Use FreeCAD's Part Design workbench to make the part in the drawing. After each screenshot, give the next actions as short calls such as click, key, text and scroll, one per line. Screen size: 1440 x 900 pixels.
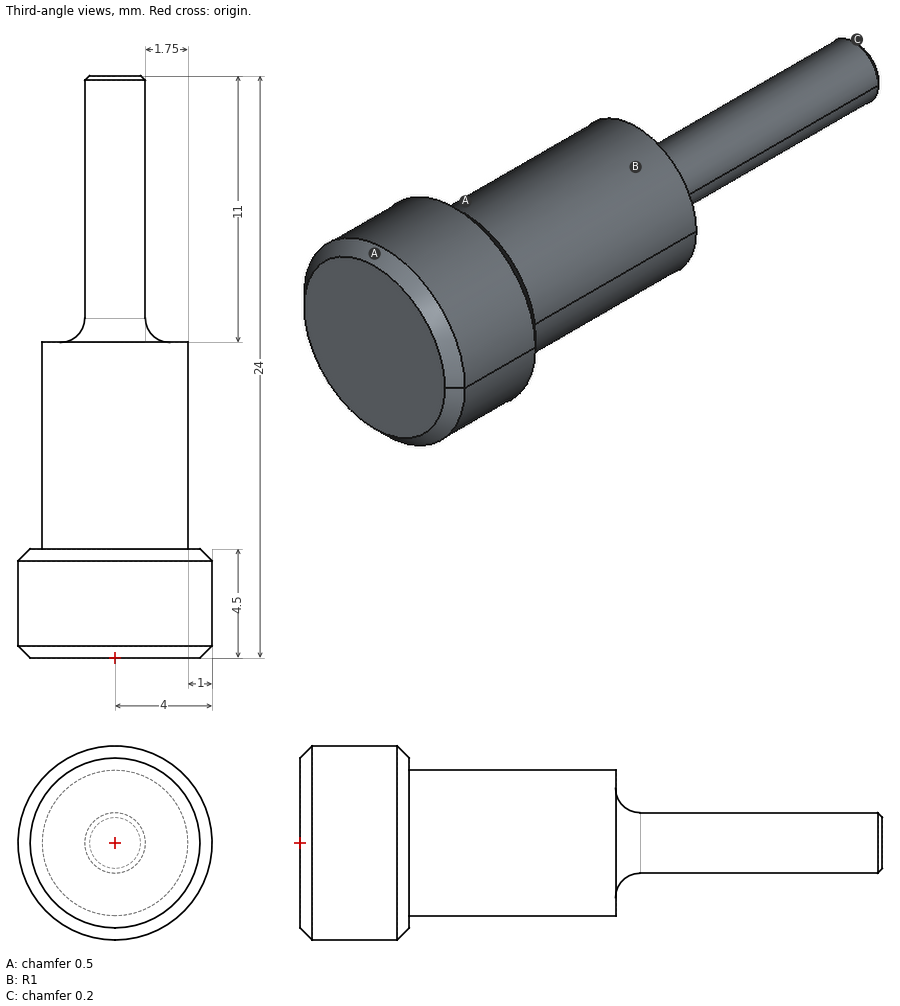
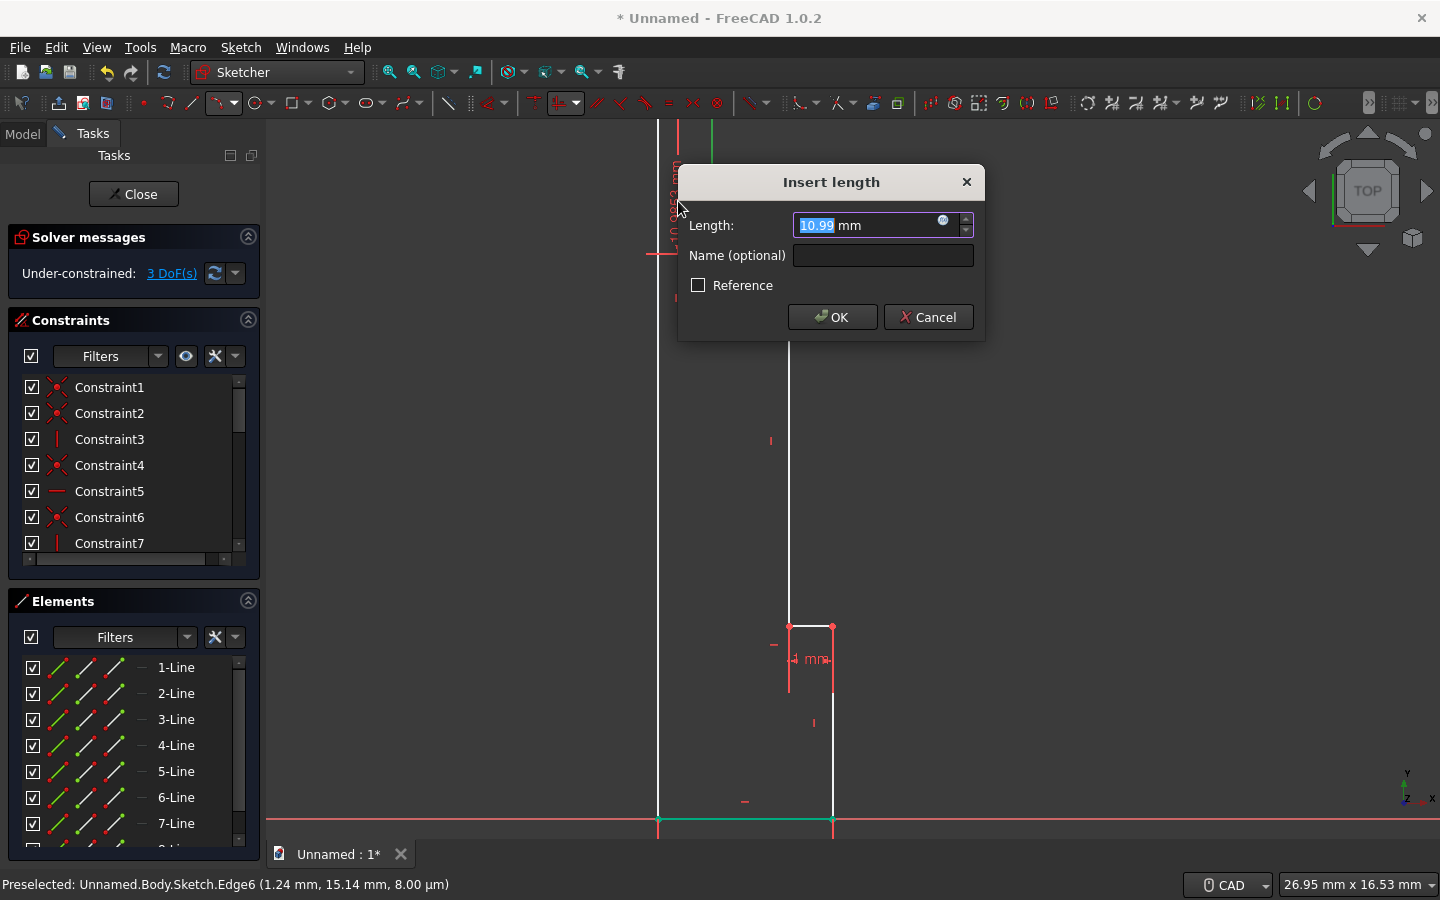
text(11)
key(Return)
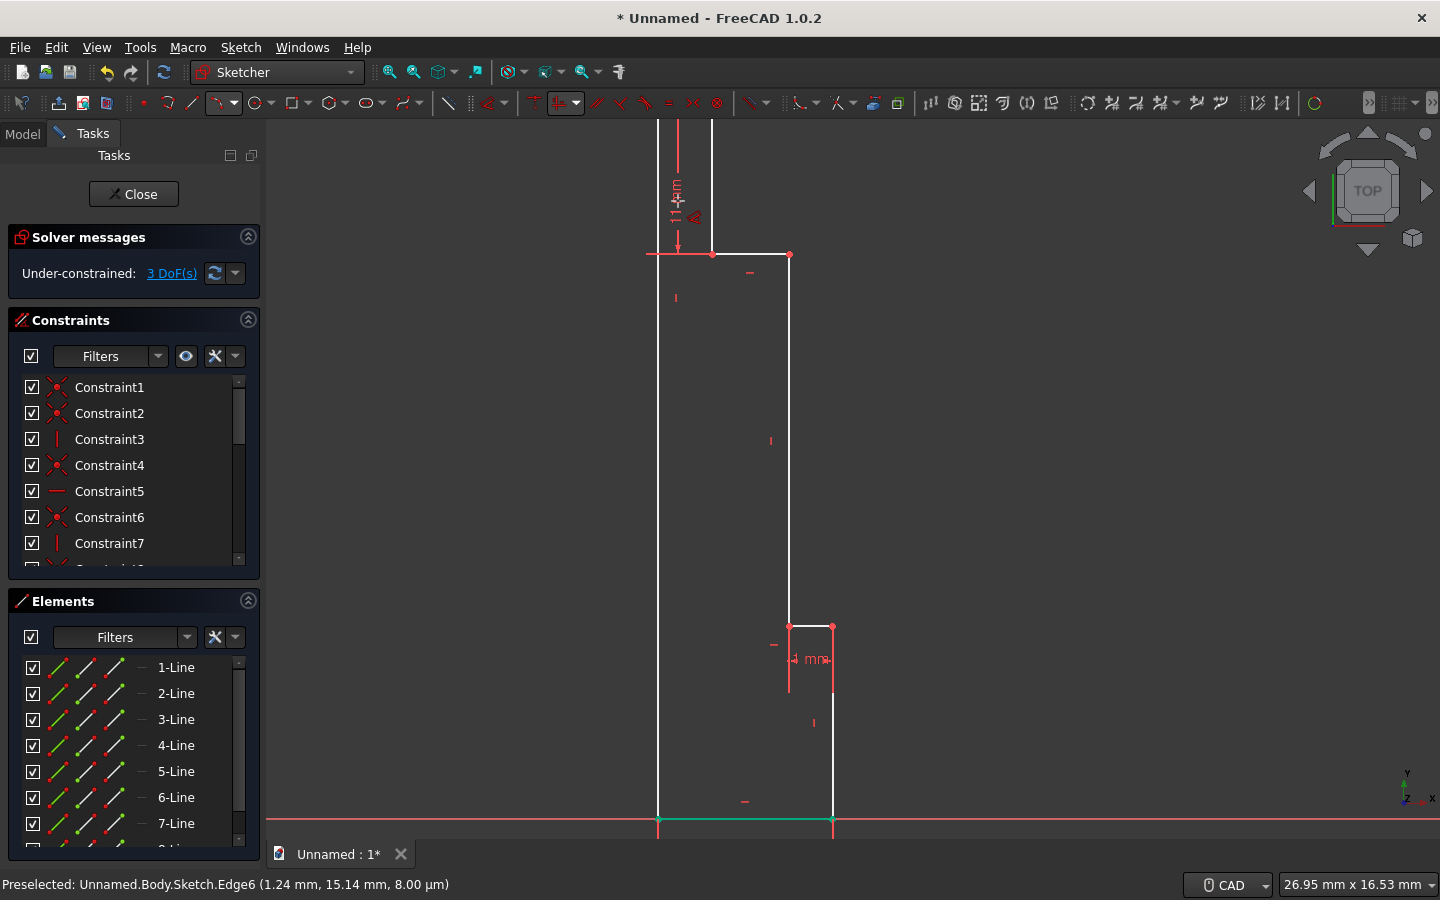
click(658, 506)
click(624, 479)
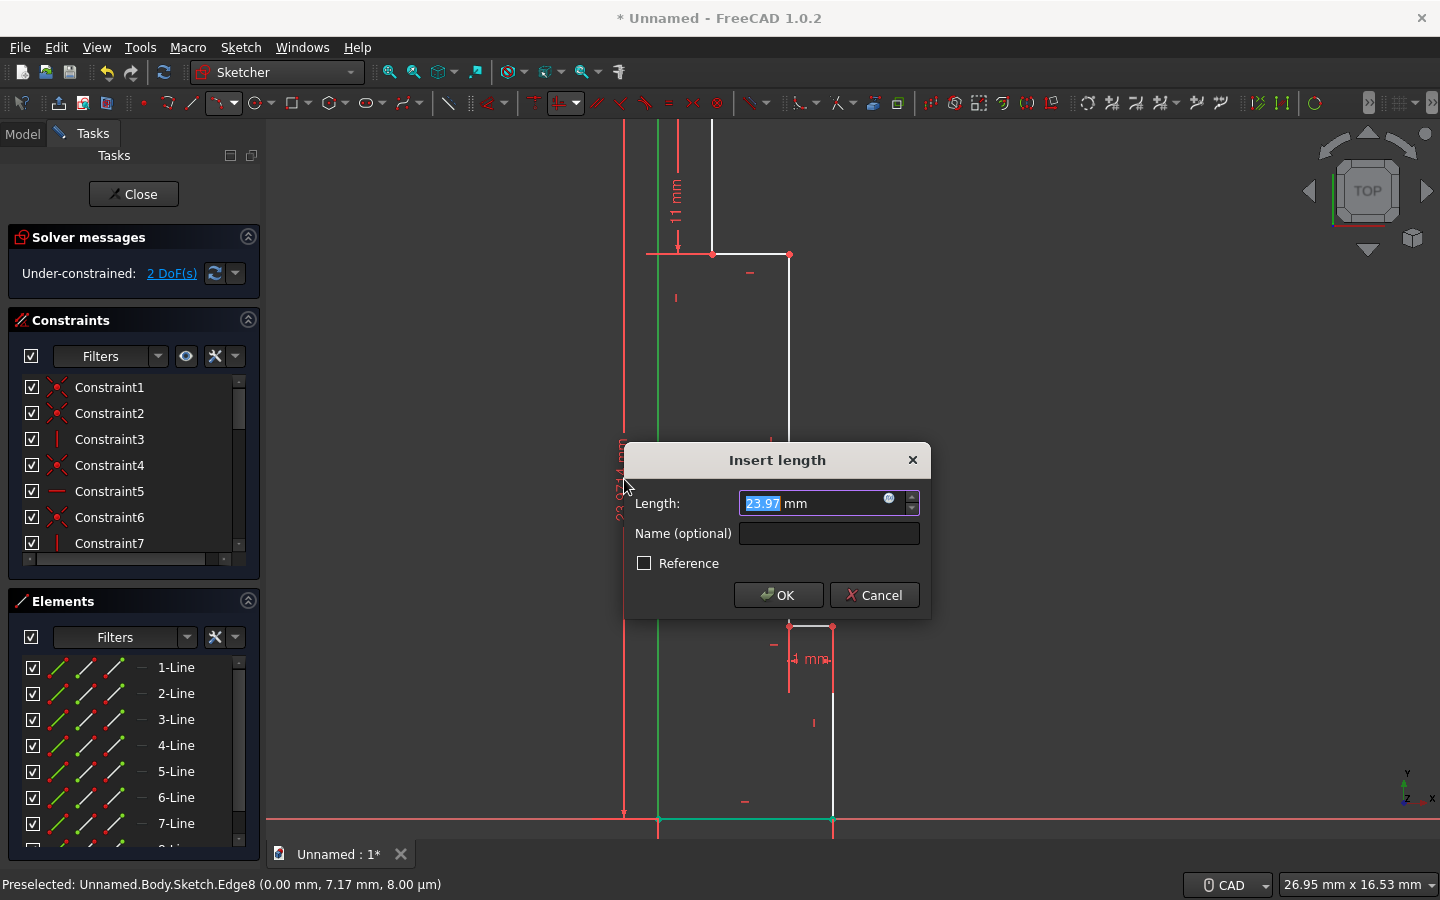
text(24)
key(Return)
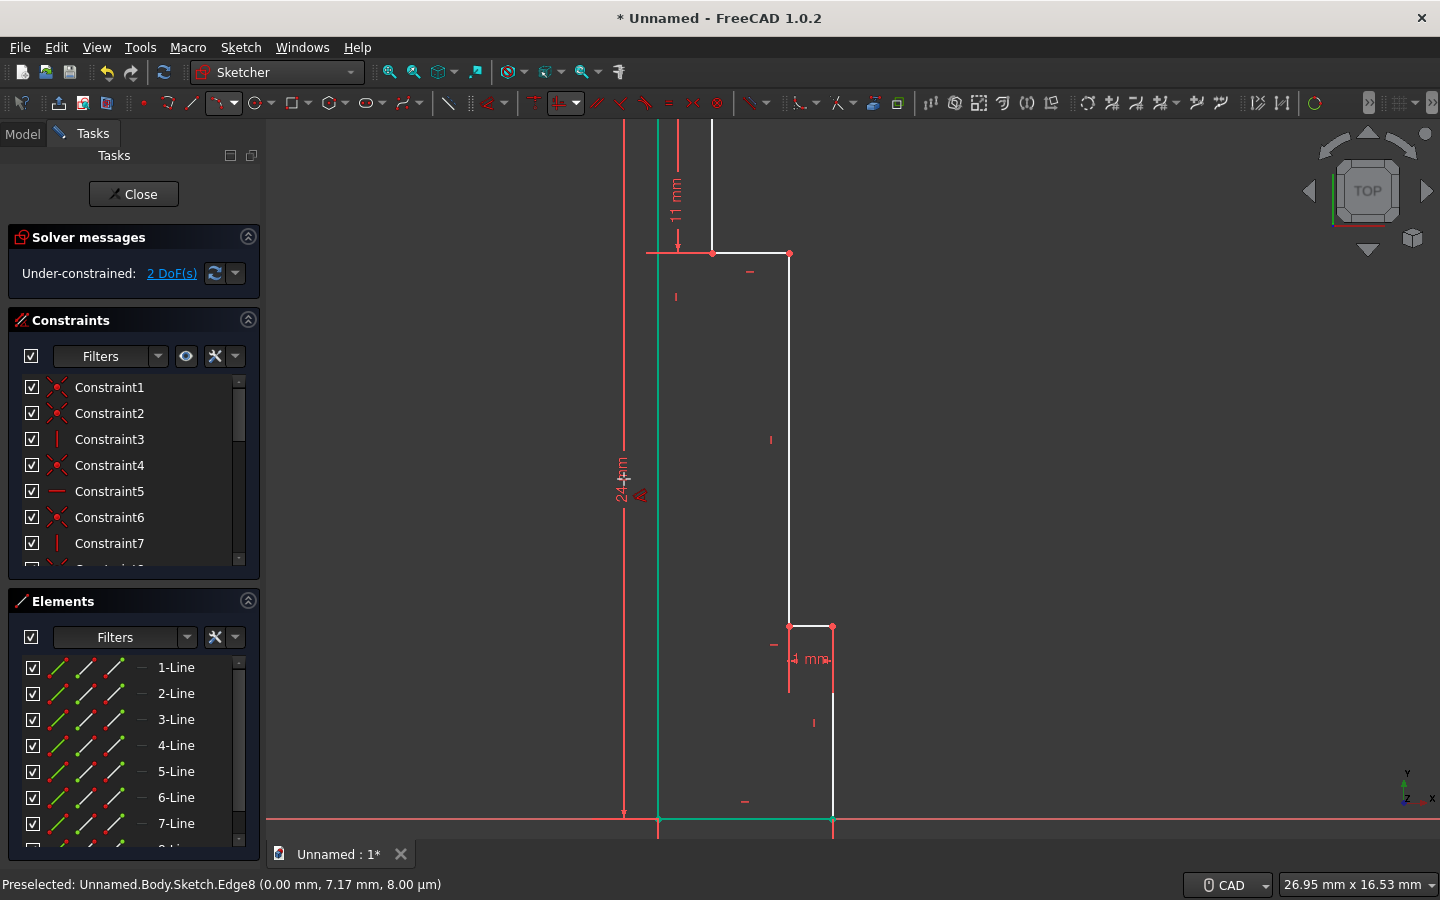
click(833, 761)
click(867, 719)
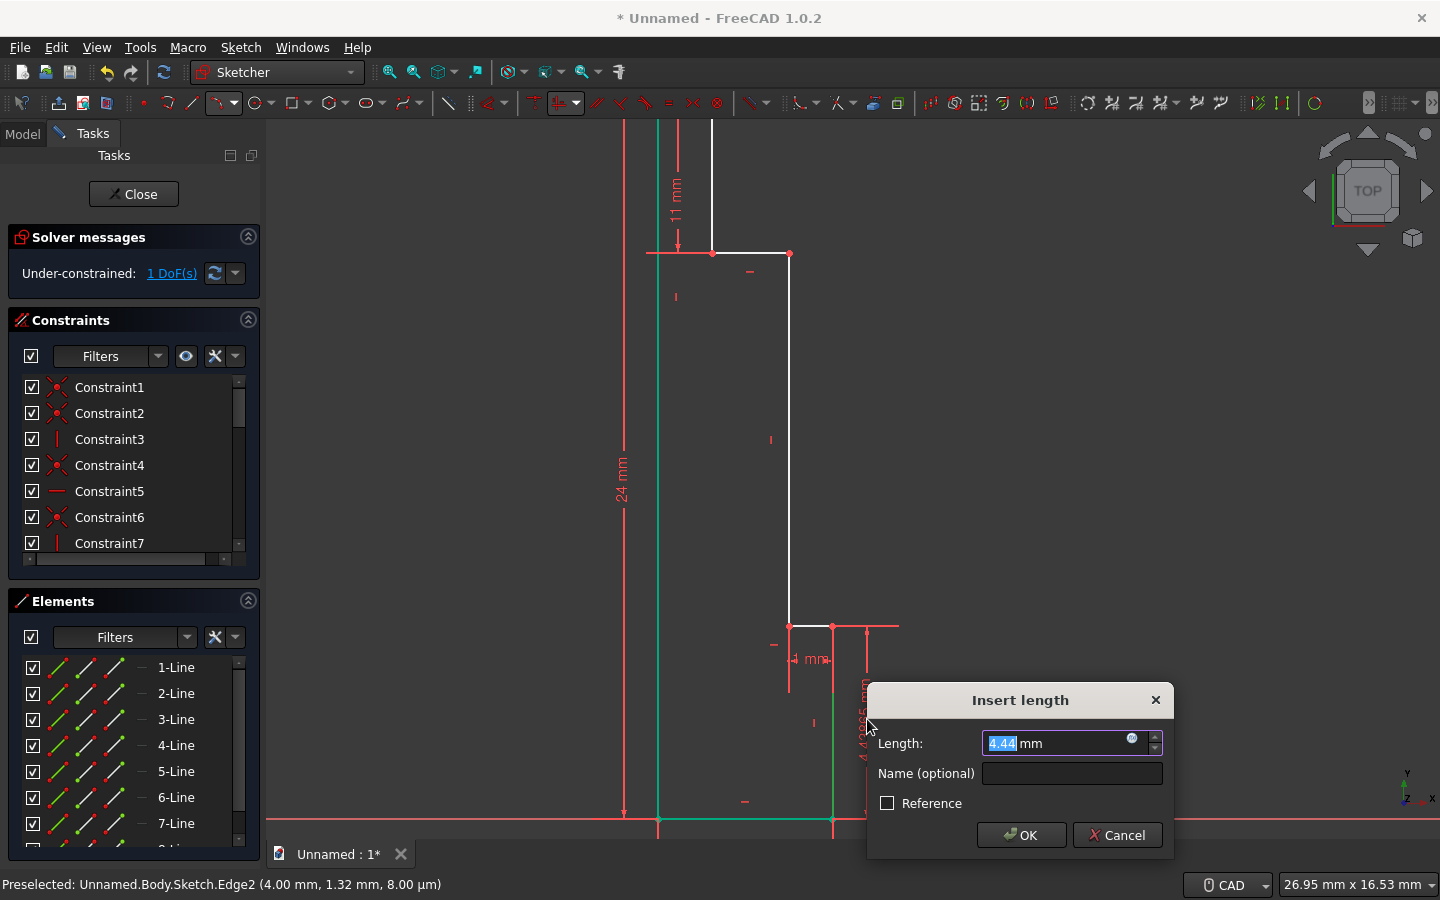
text(4.5)
key(Return)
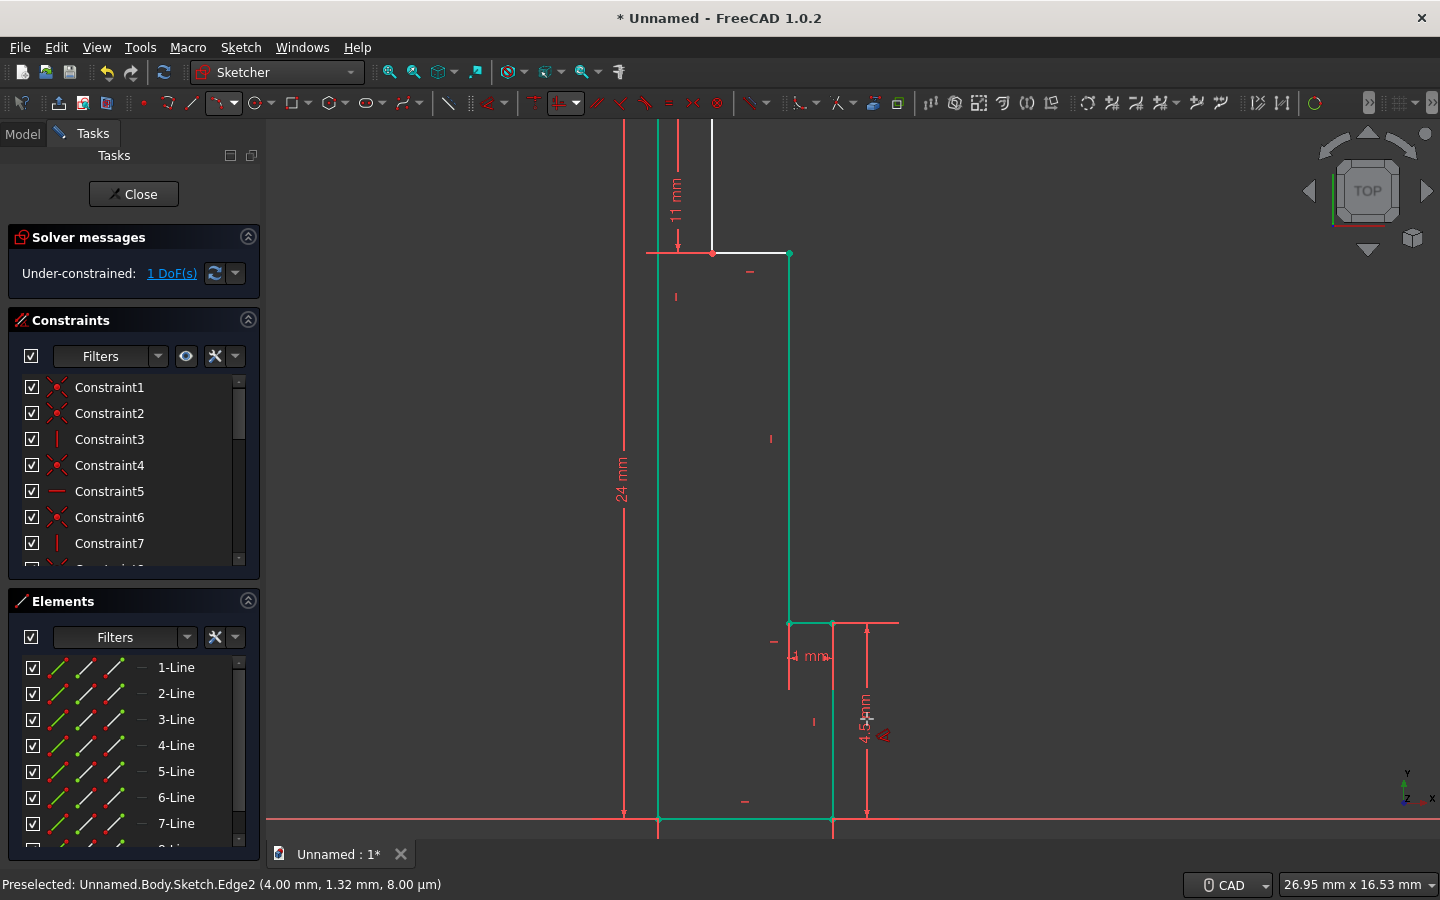
click(766, 253)
click(751, 219)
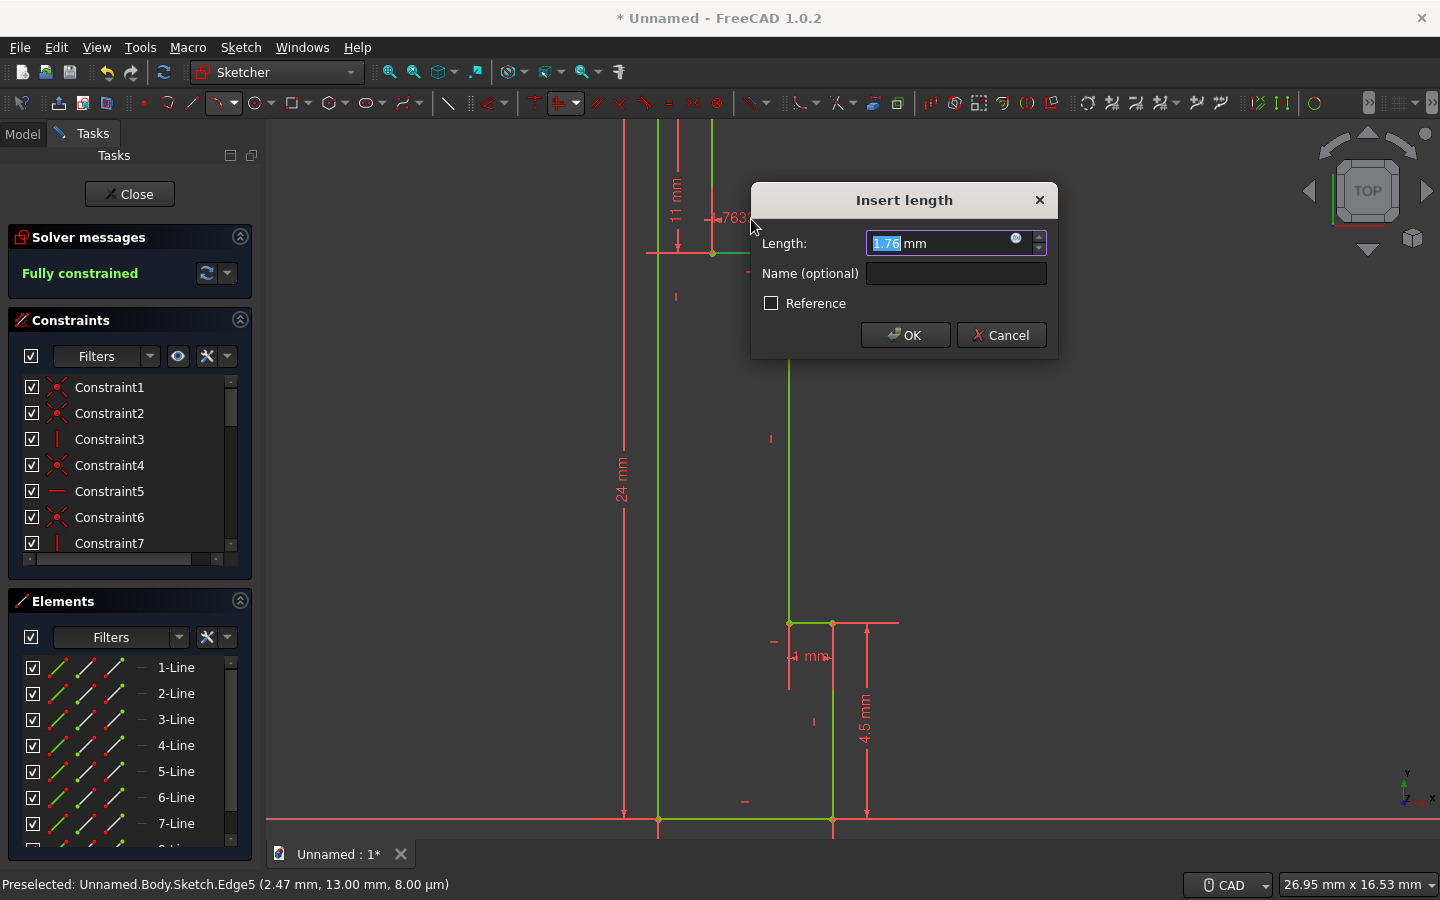
text(1.75)
key(Return)
key(Escape)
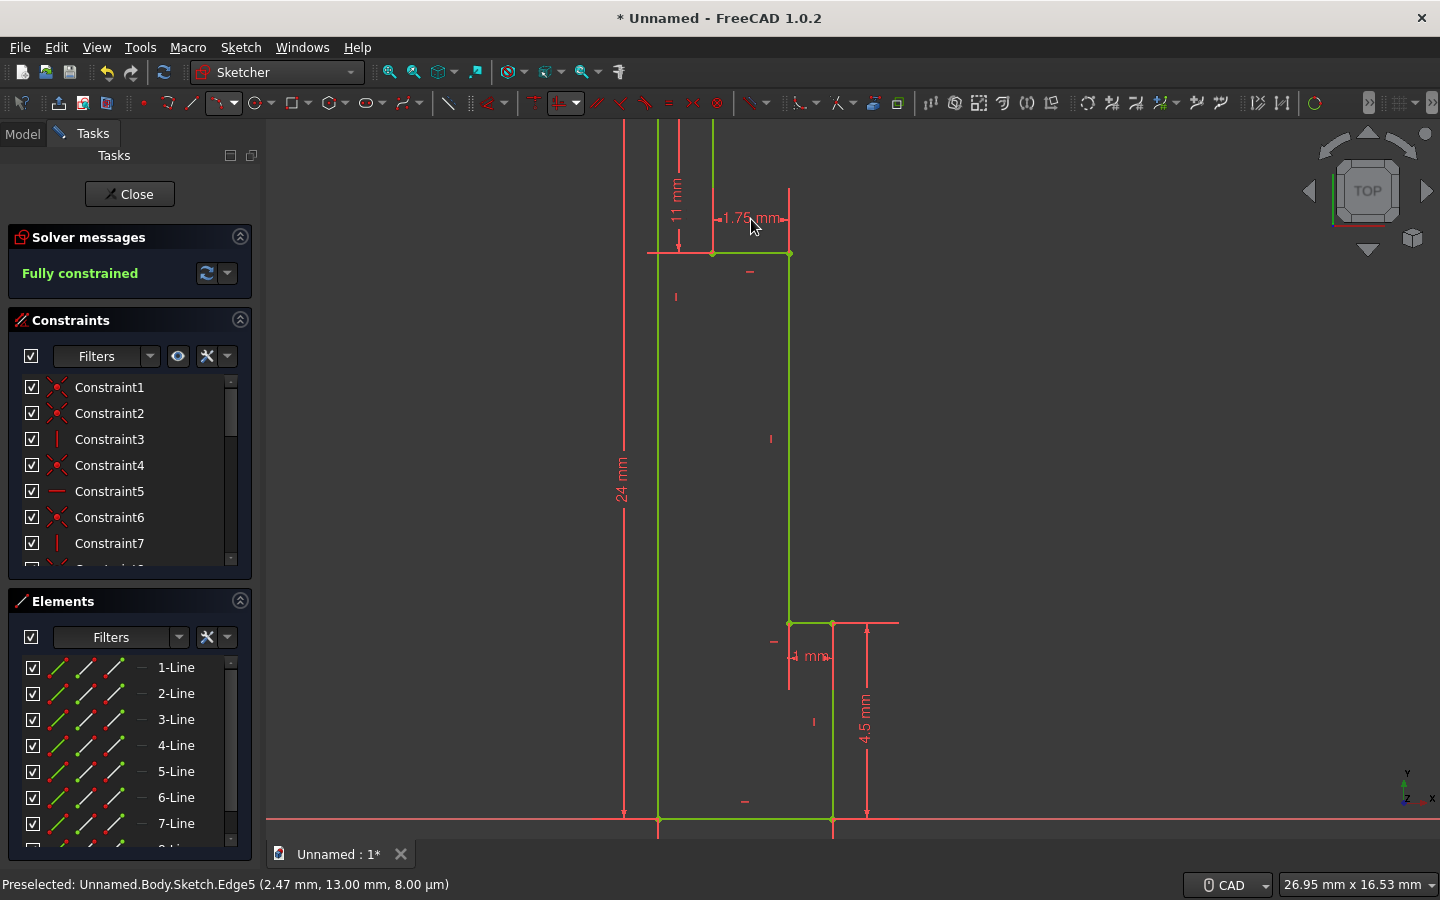
click(130, 194)